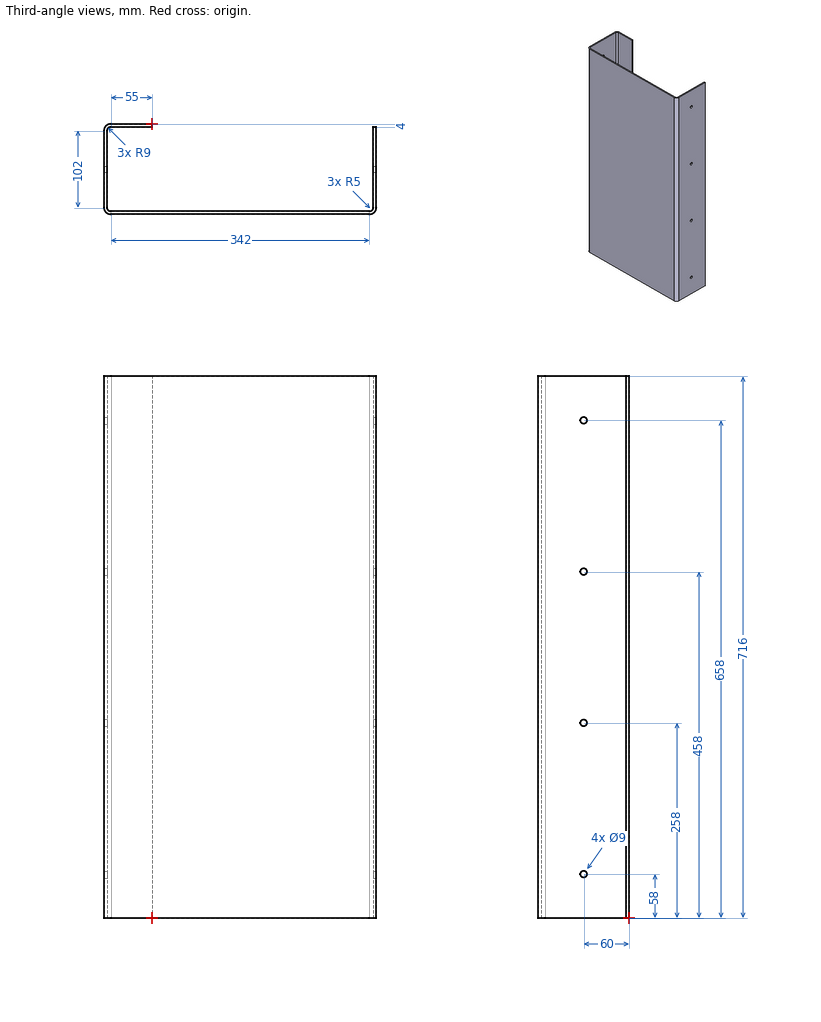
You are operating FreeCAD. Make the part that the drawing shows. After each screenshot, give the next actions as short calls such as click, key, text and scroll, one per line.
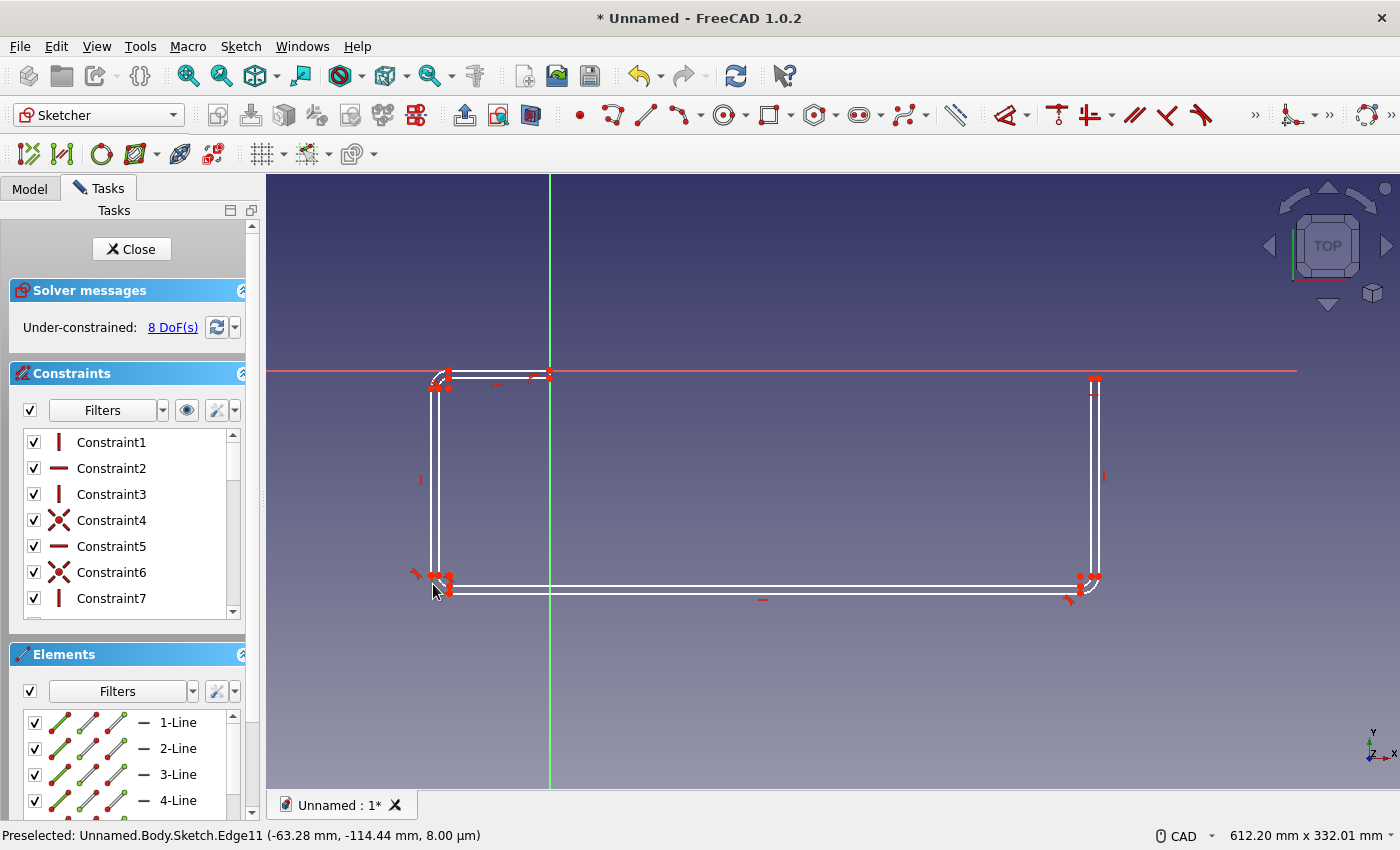
scroll(1089, 592, up, 4)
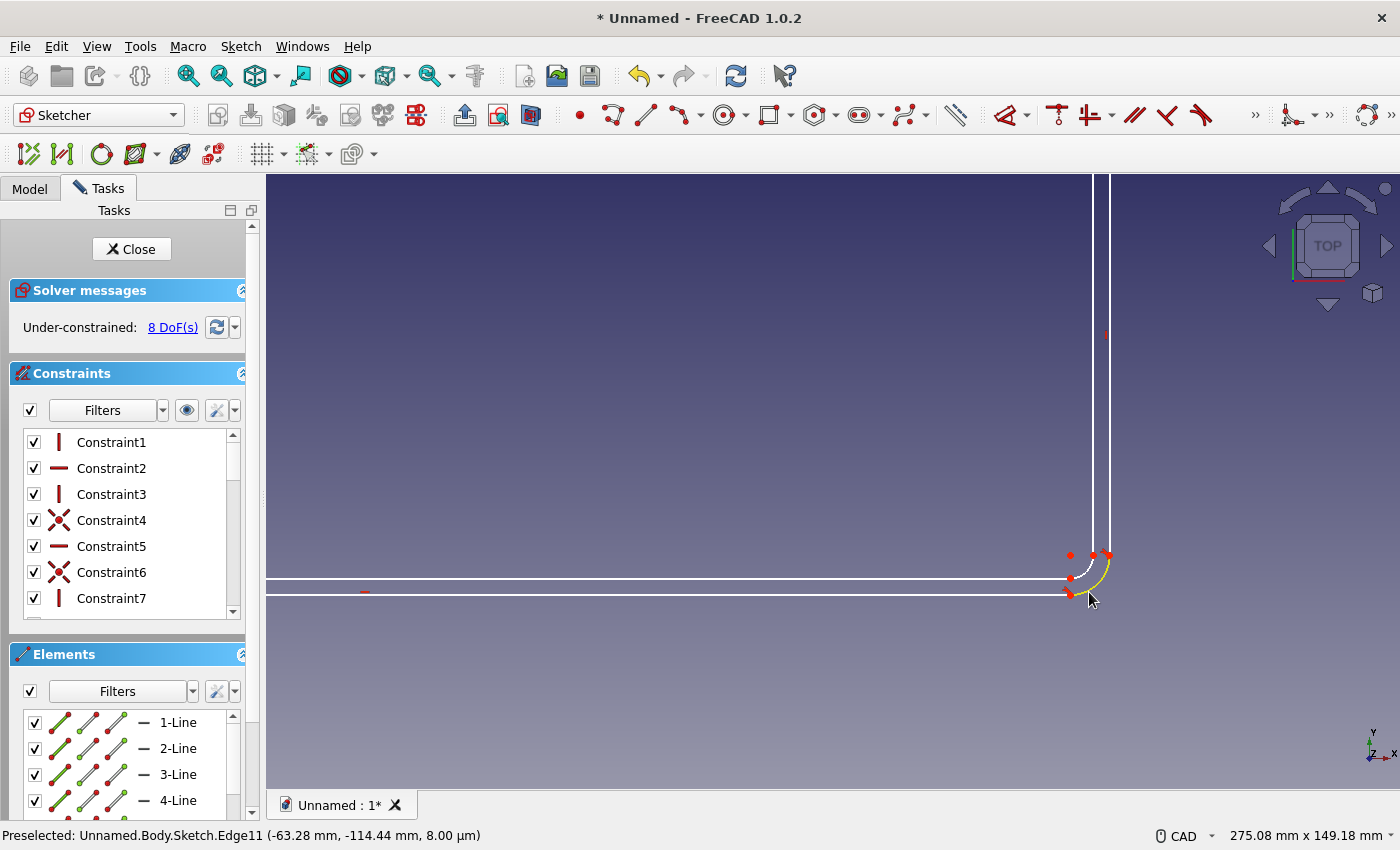
click(1088, 591)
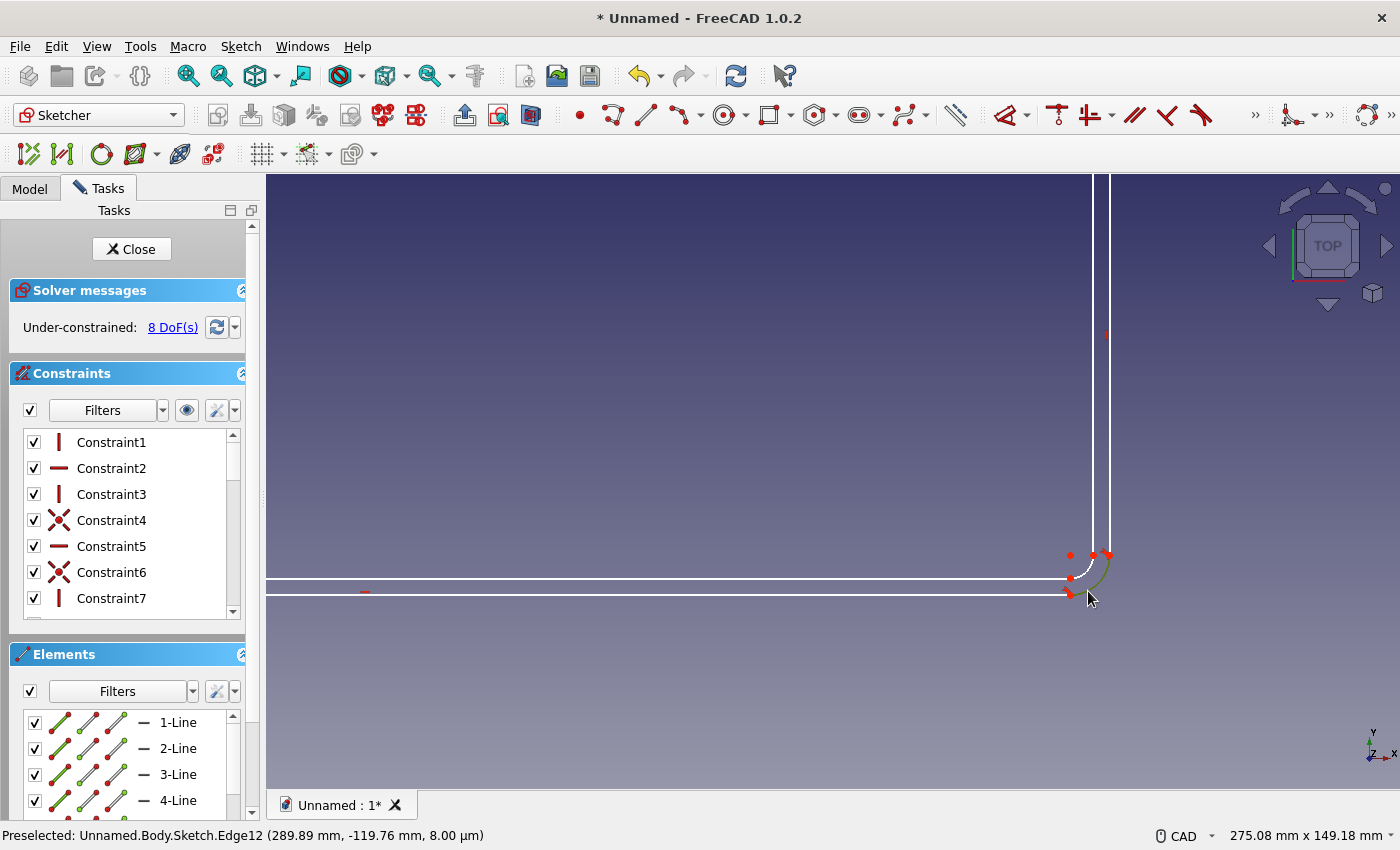
scroll(1089, 592, down, 4)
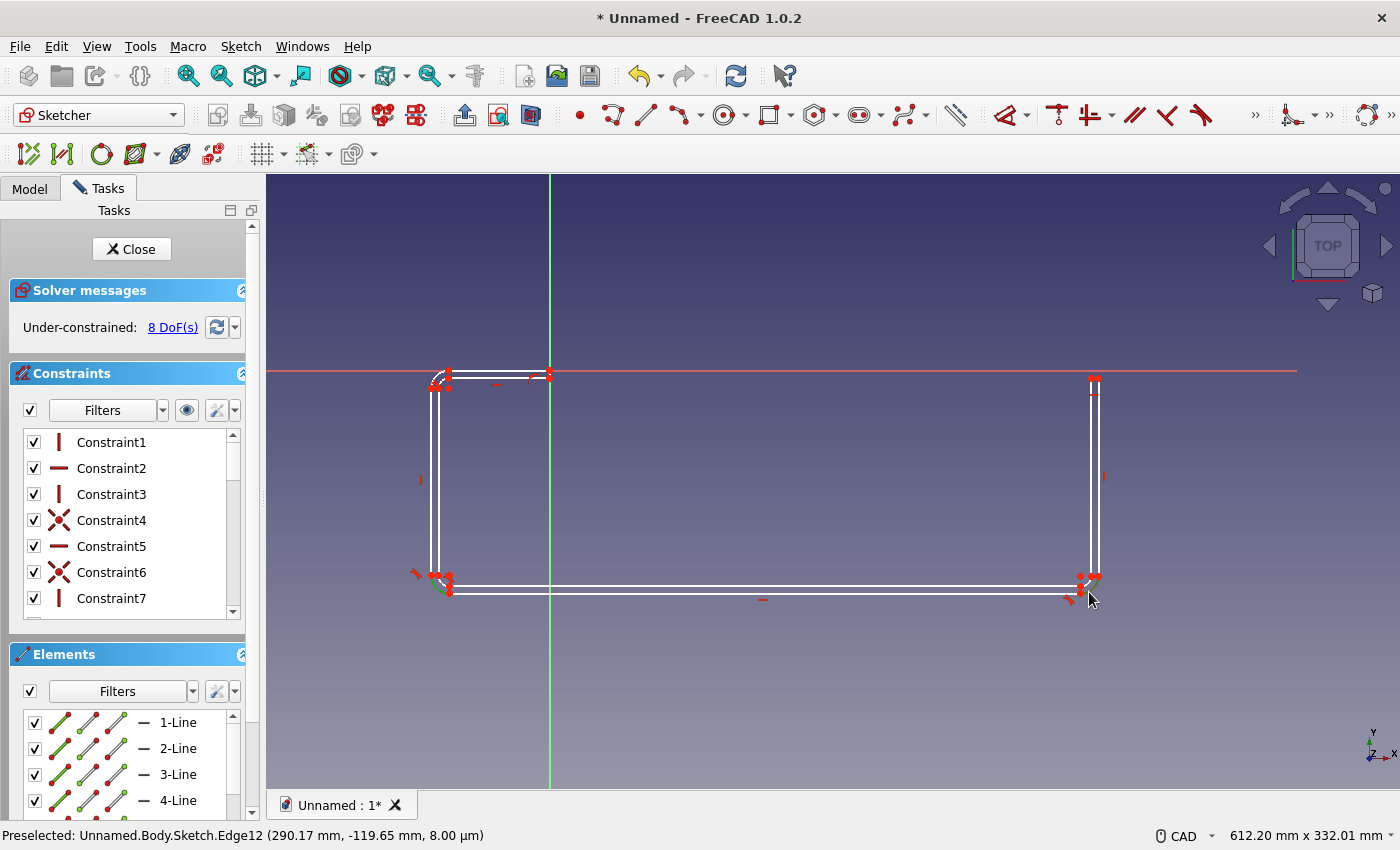
scroll(433, 380, up, 4)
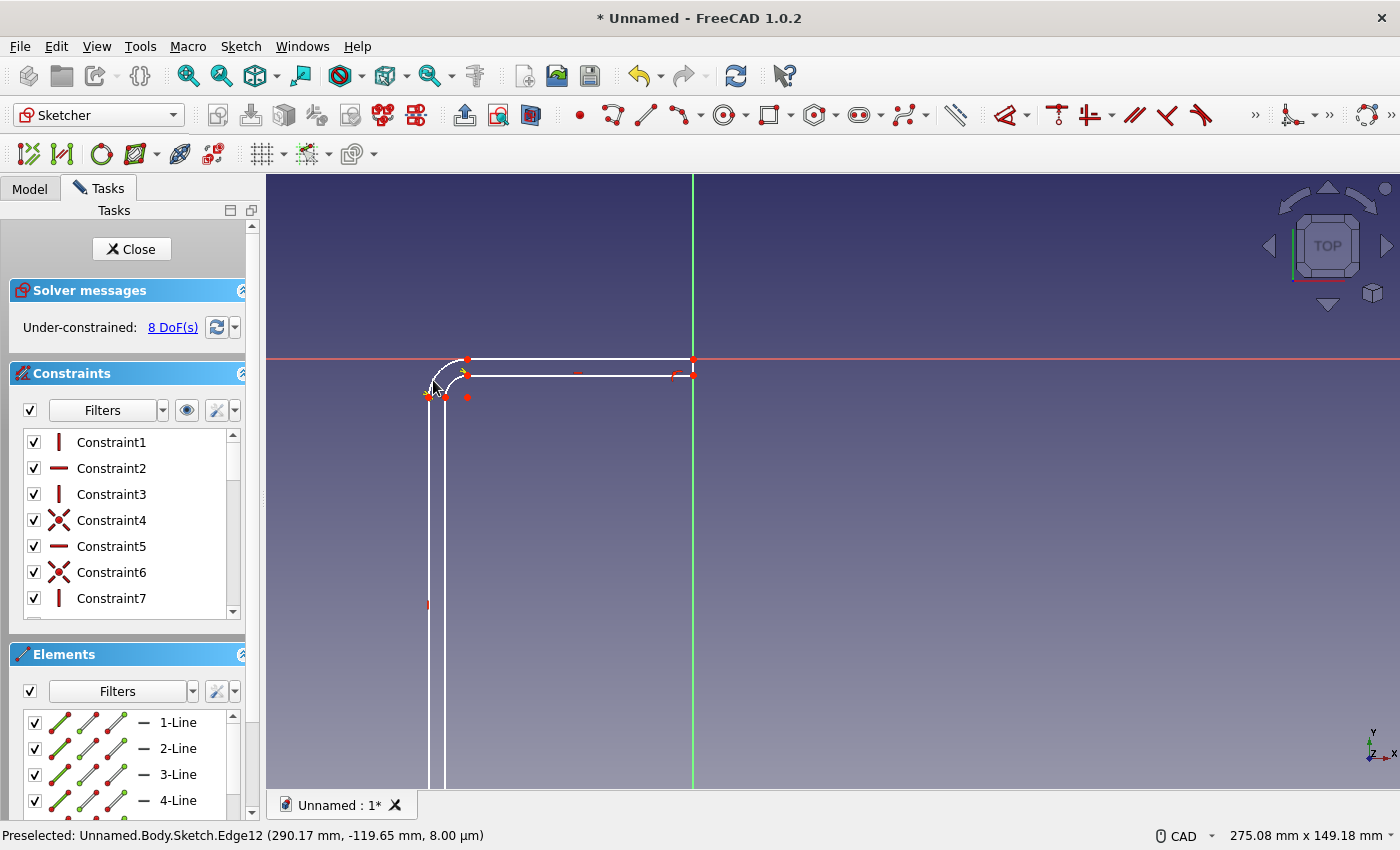
click(433, 380)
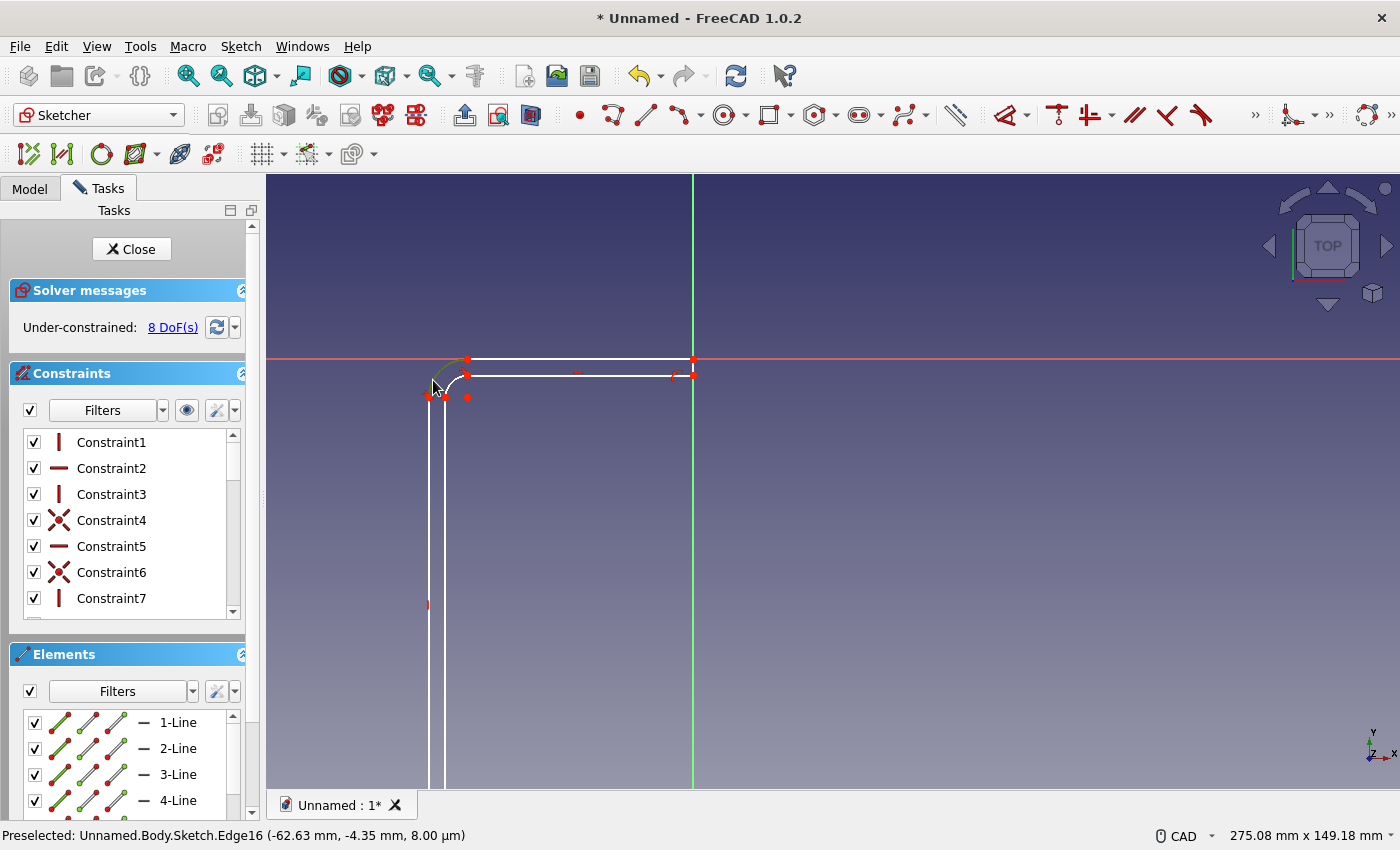
key(e)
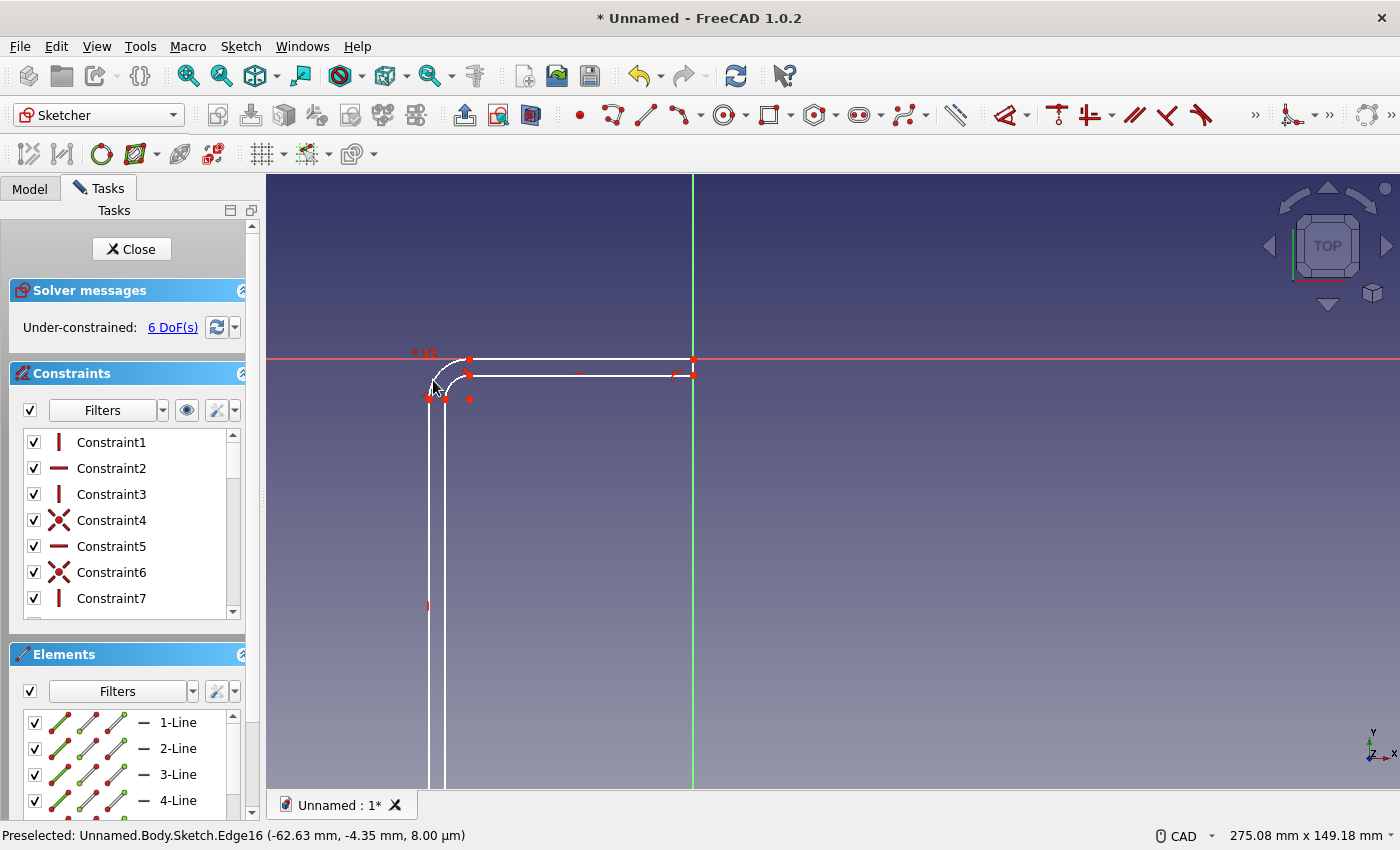
click(1004, 116)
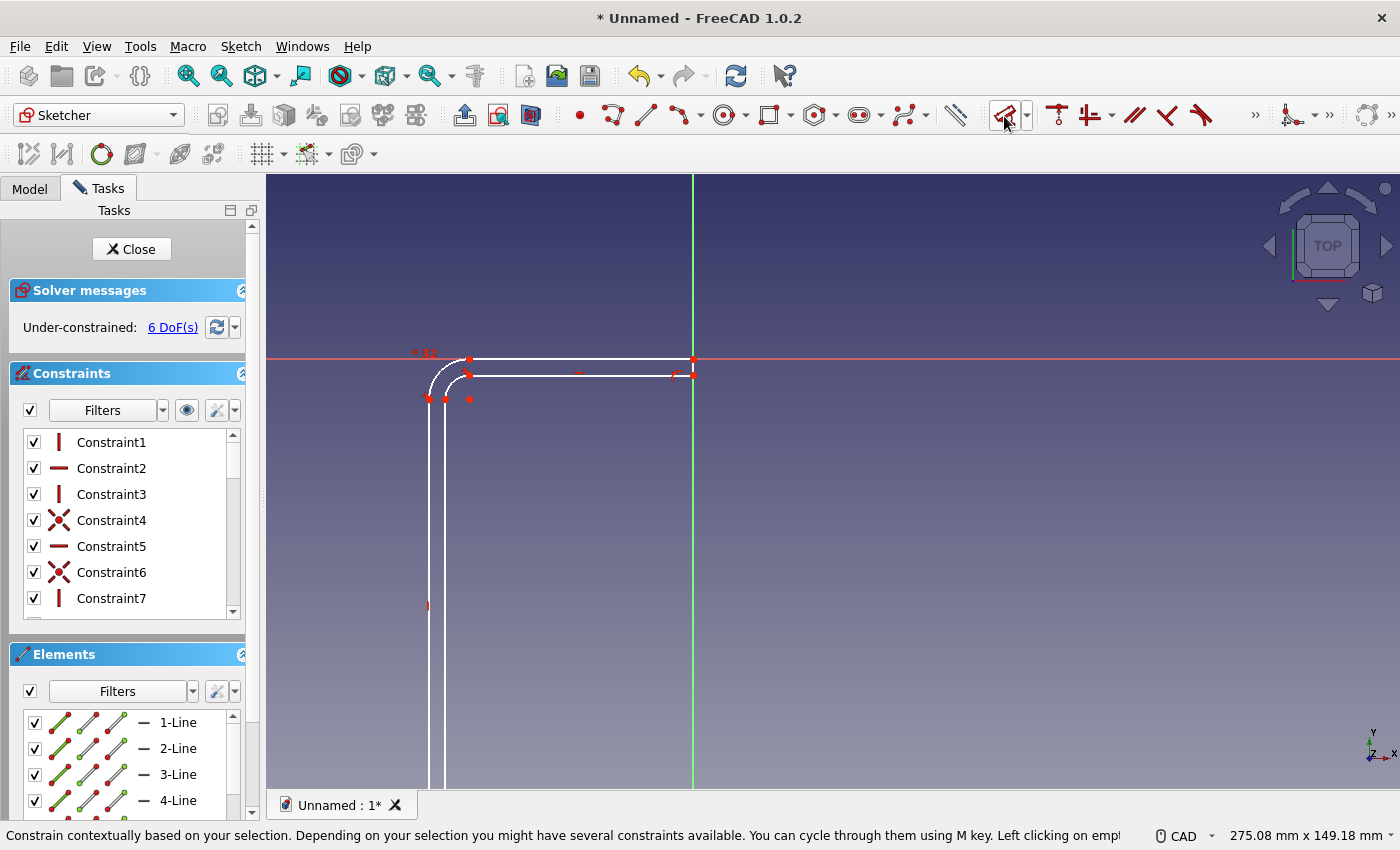
scroll(433, 379, down, 4)